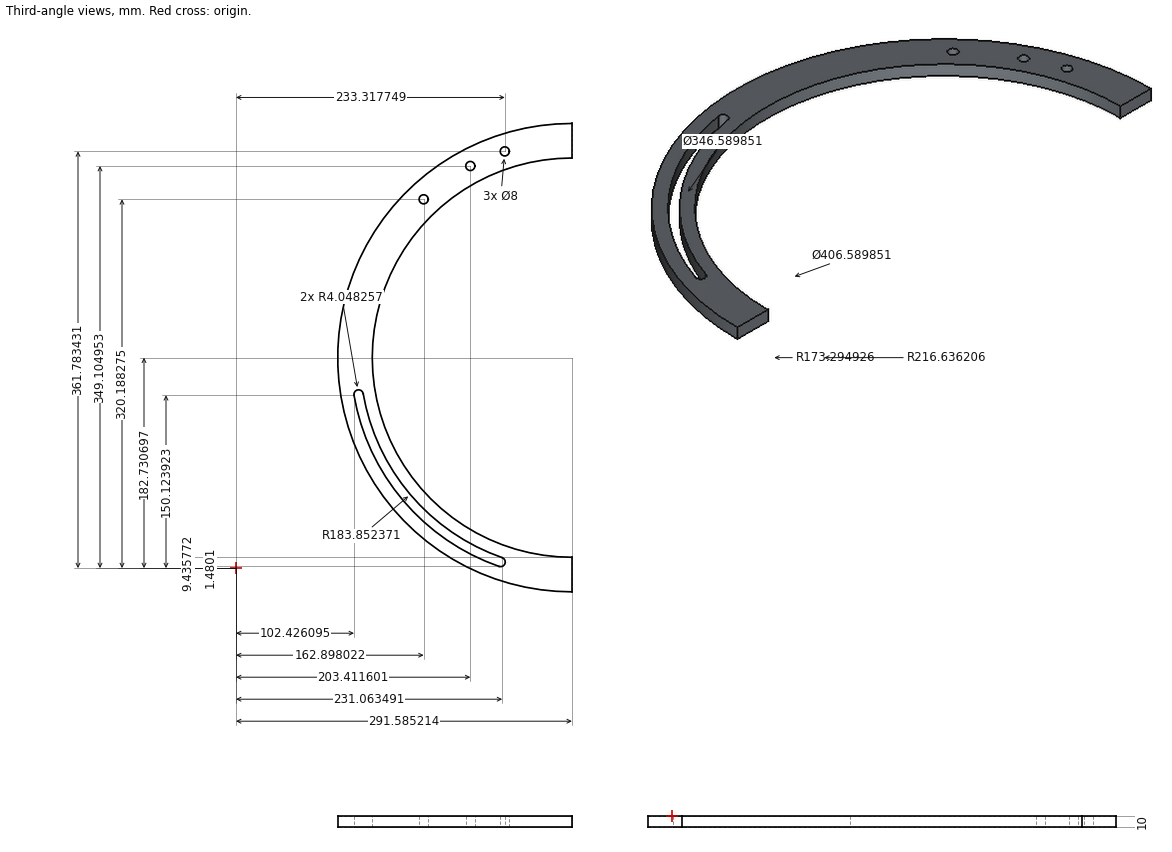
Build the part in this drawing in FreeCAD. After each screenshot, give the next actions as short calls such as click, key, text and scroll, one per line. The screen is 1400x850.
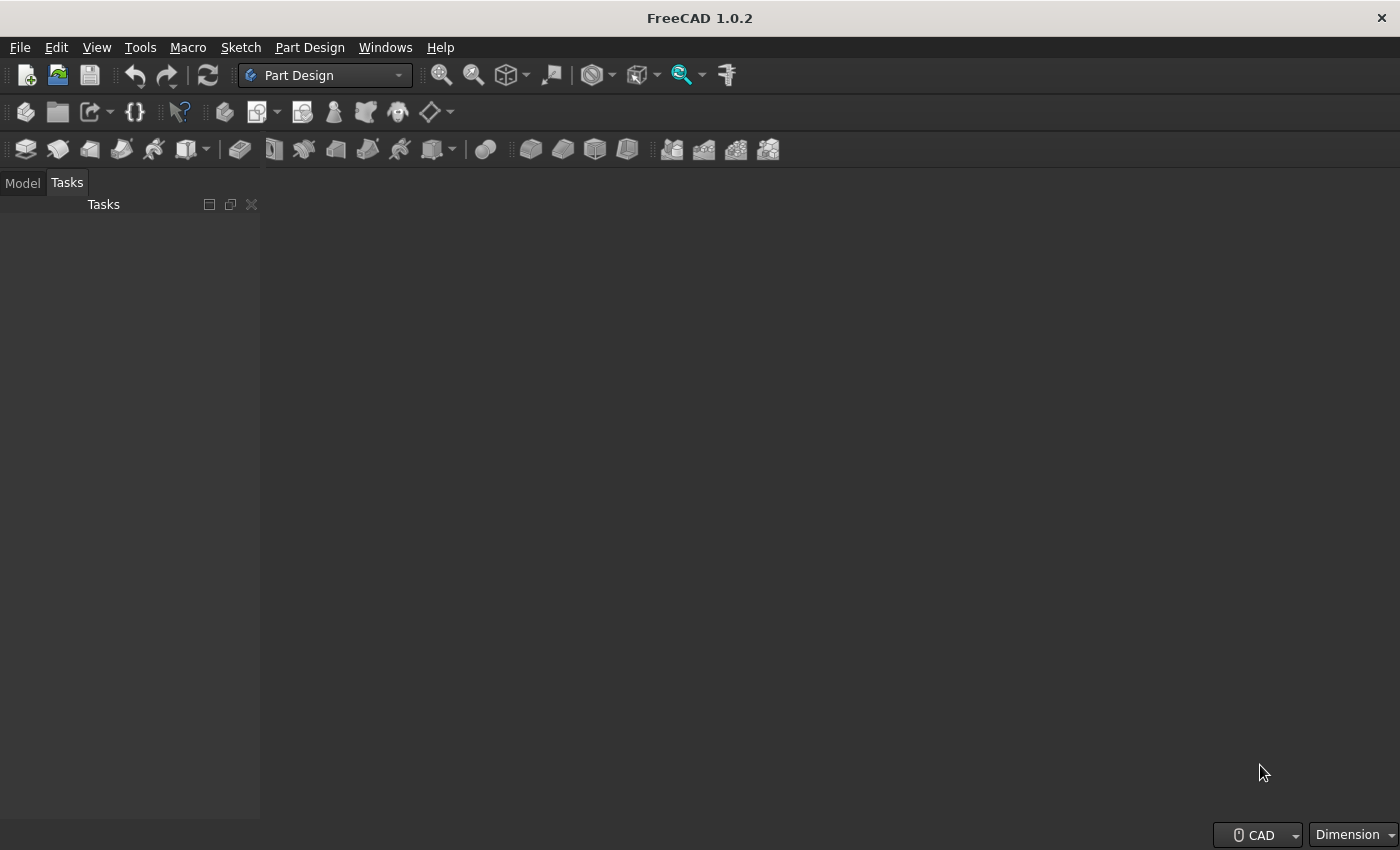
click(498, 76)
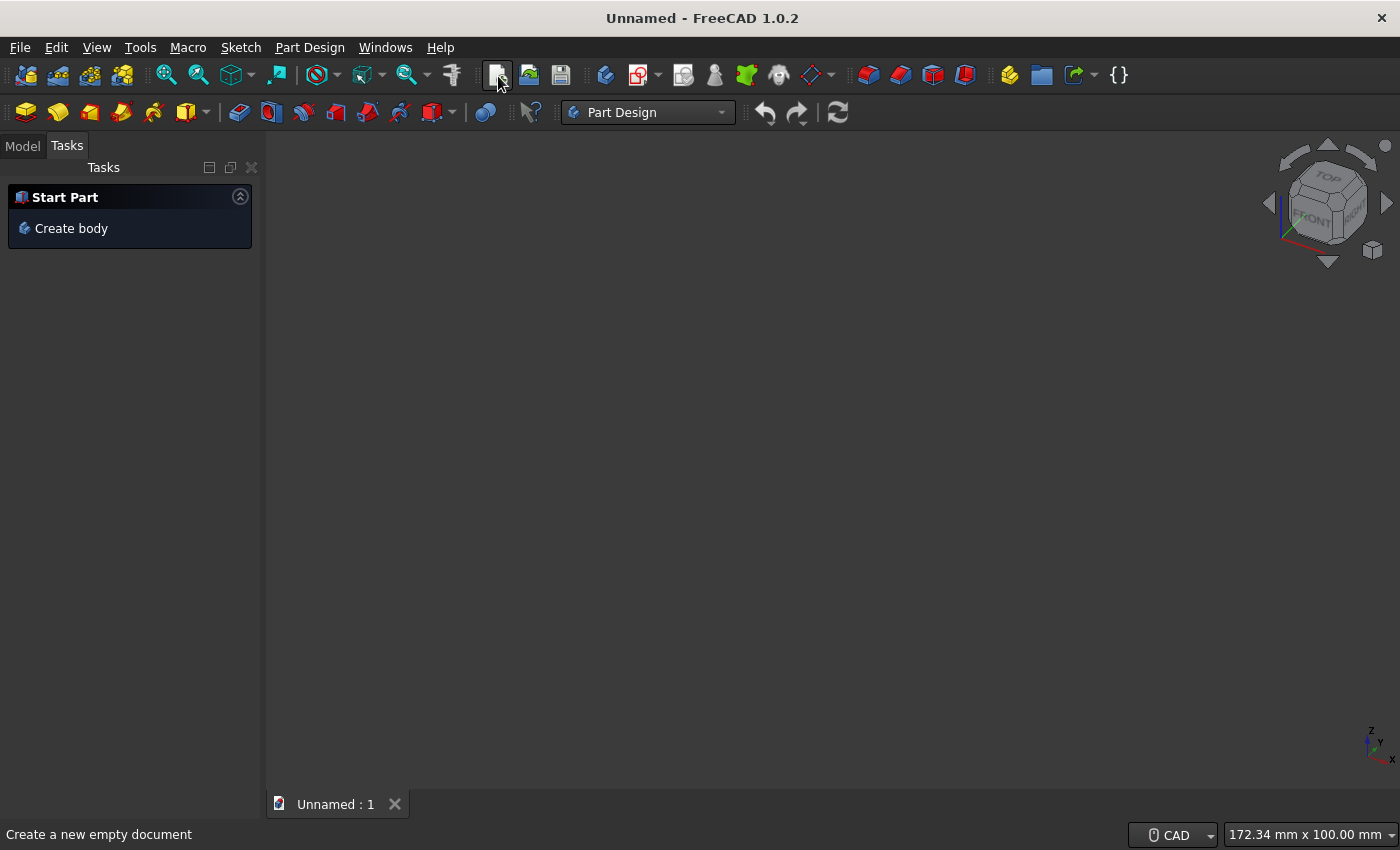
click(638, 76)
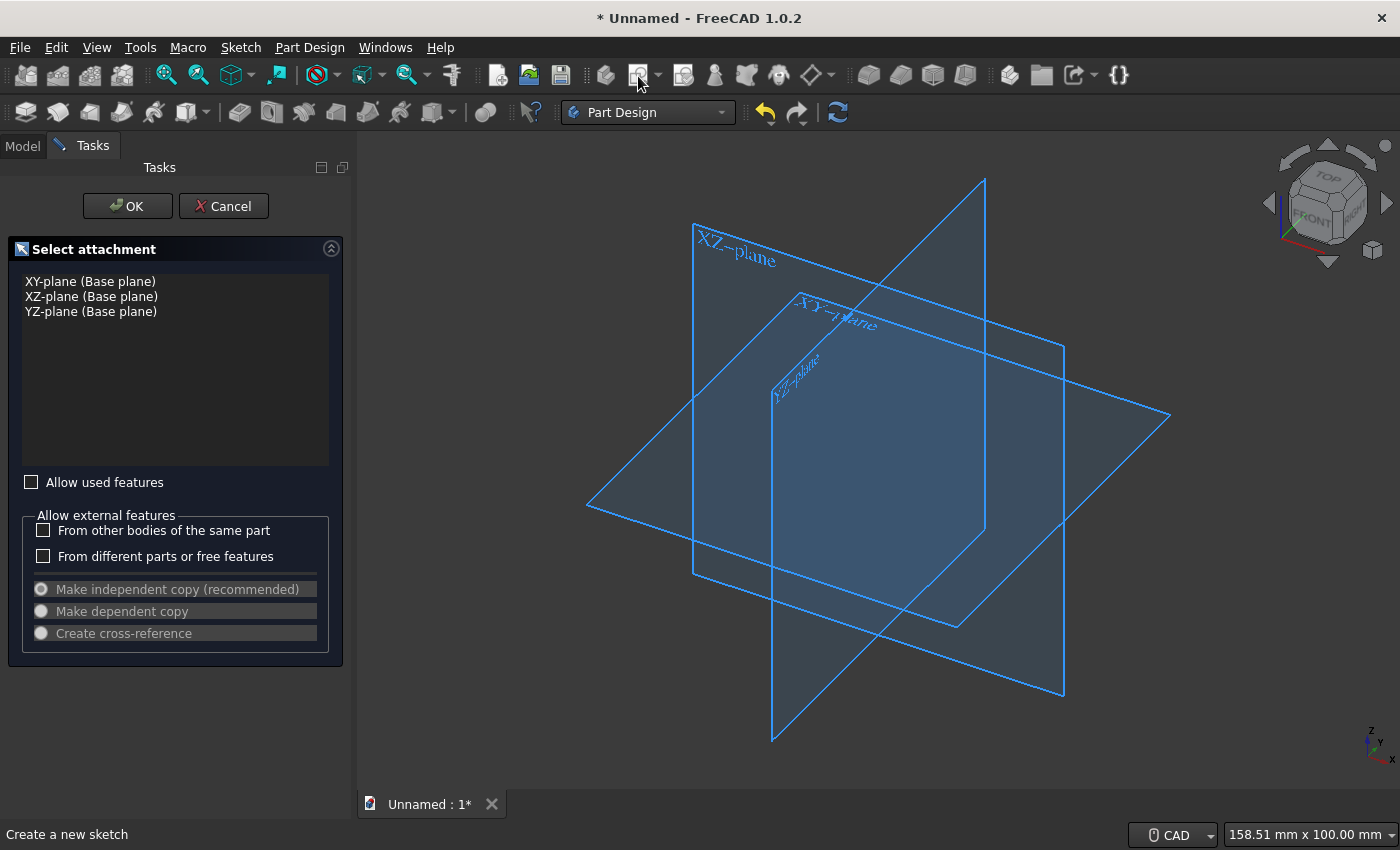
click(82, 282)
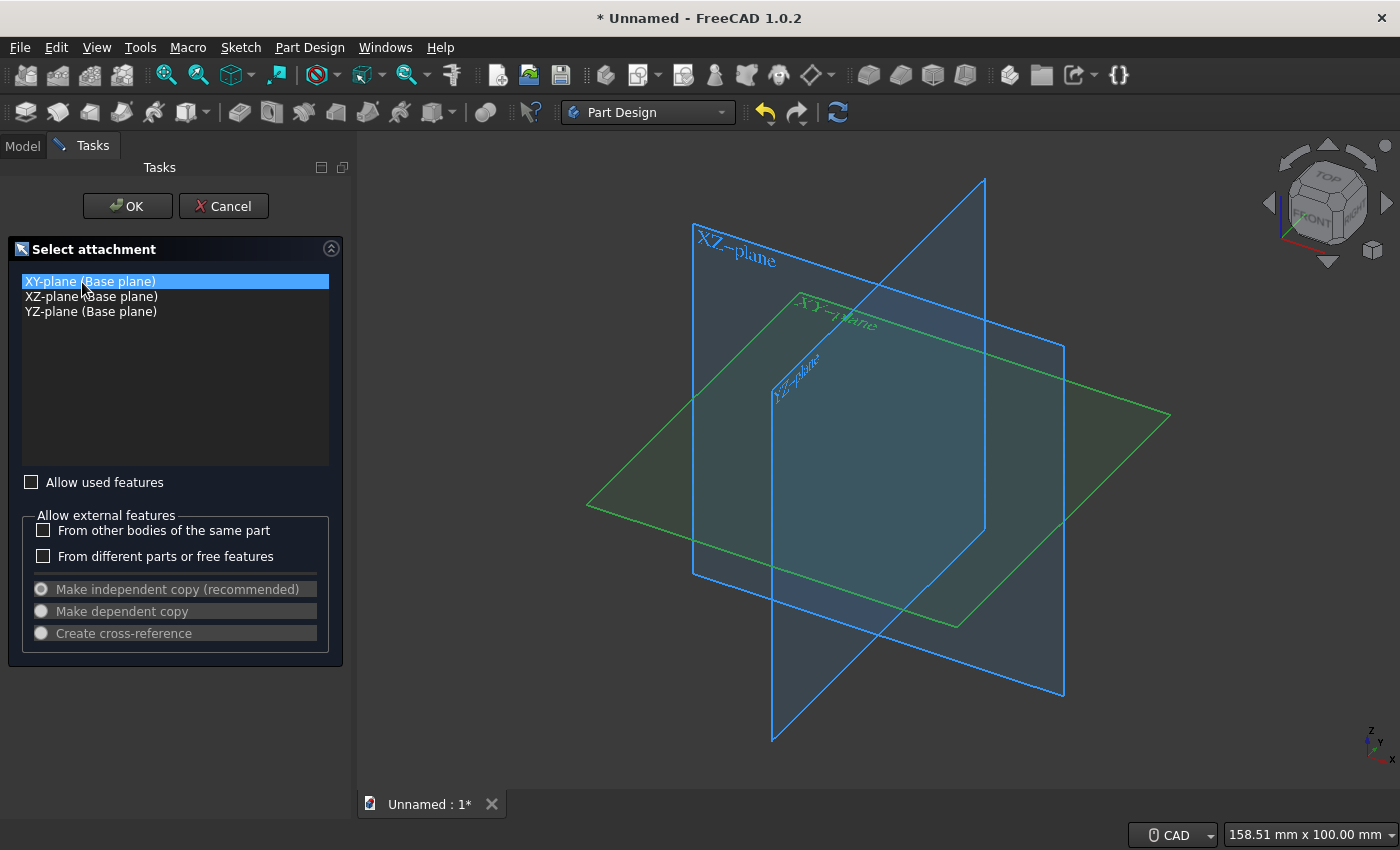
click(128, 206)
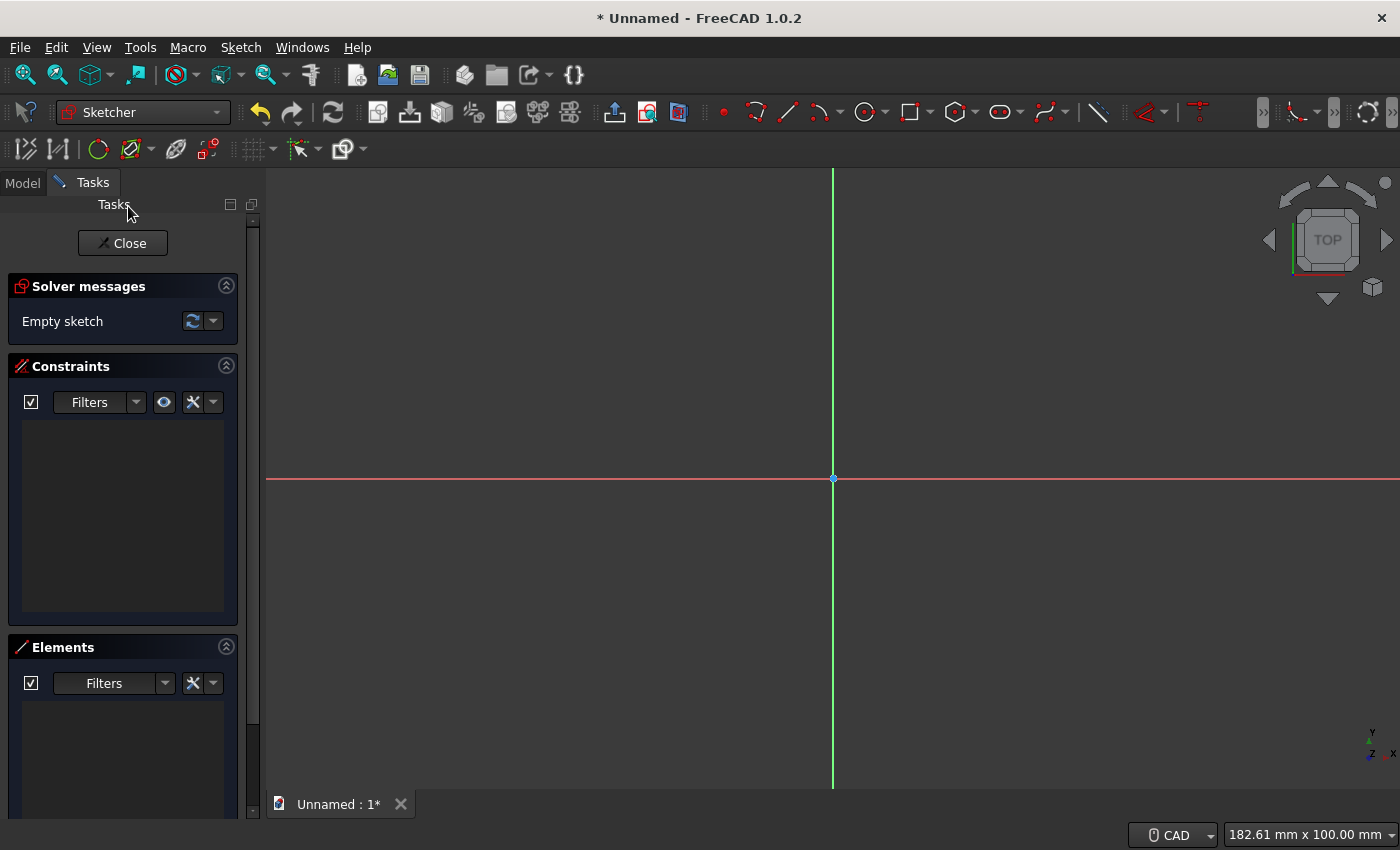
scroll(447, 703, down, 9)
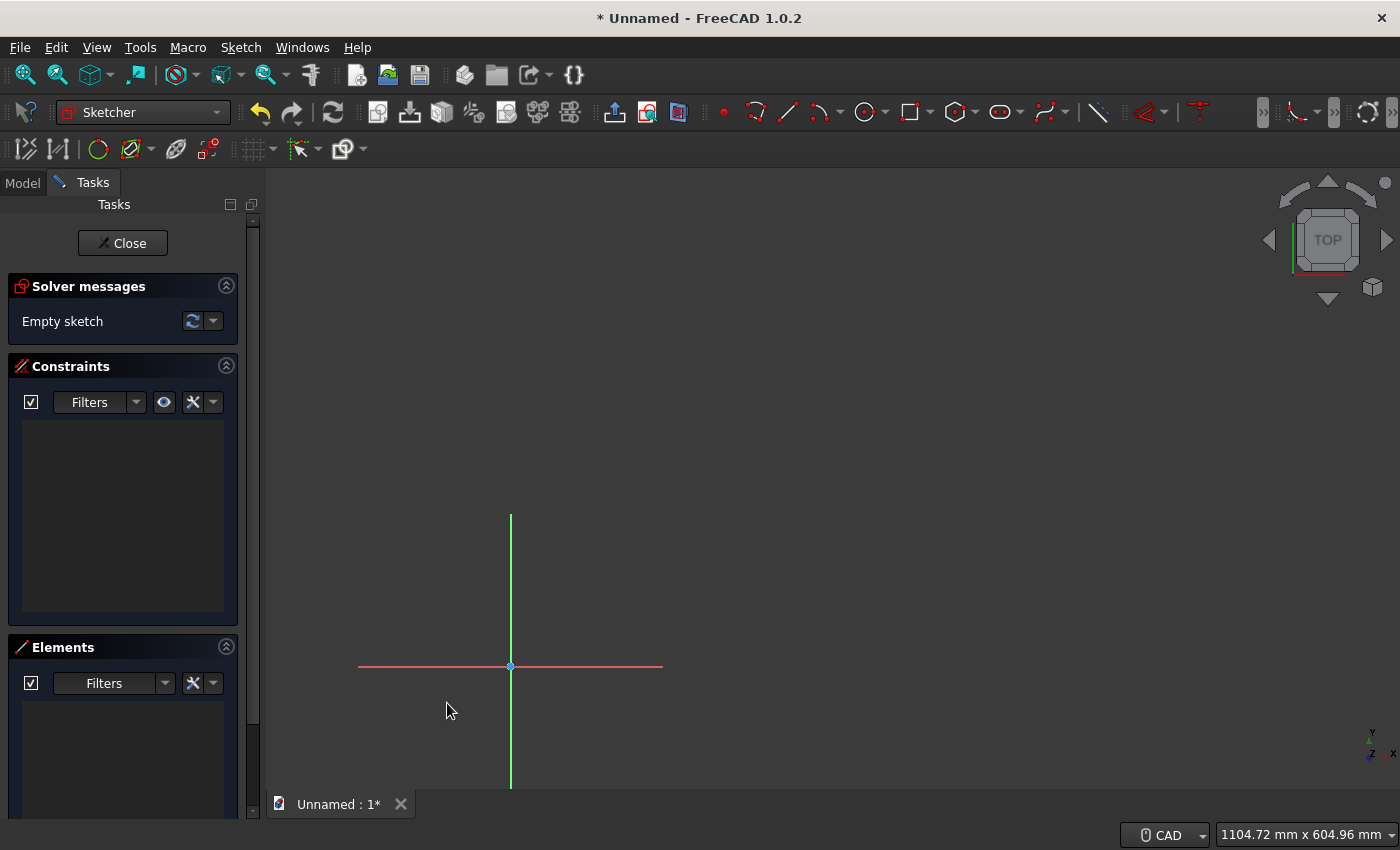
click(866, 112)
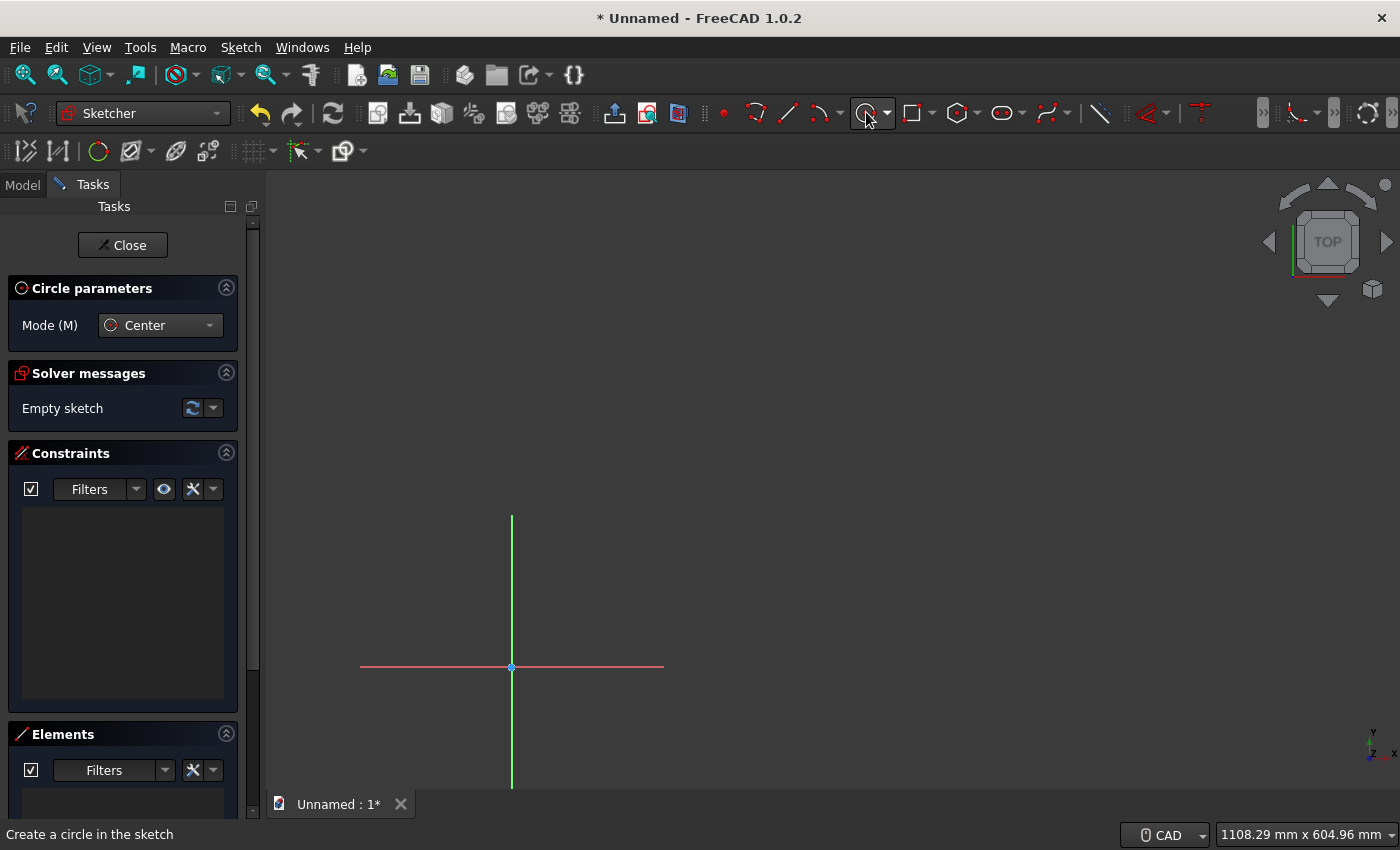
click(810, 480)
move(957, 333)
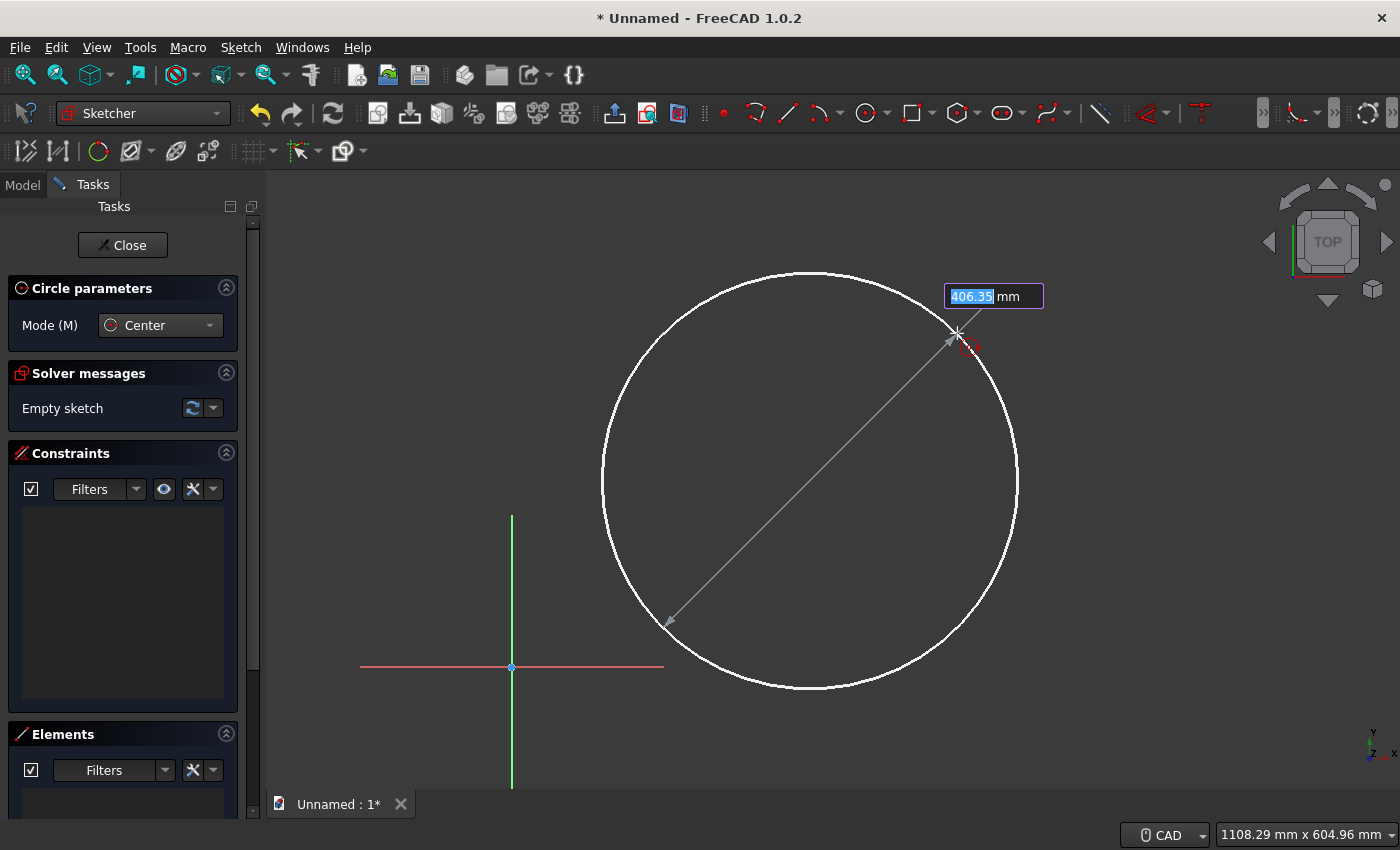
text(406.589851)
key(Return)